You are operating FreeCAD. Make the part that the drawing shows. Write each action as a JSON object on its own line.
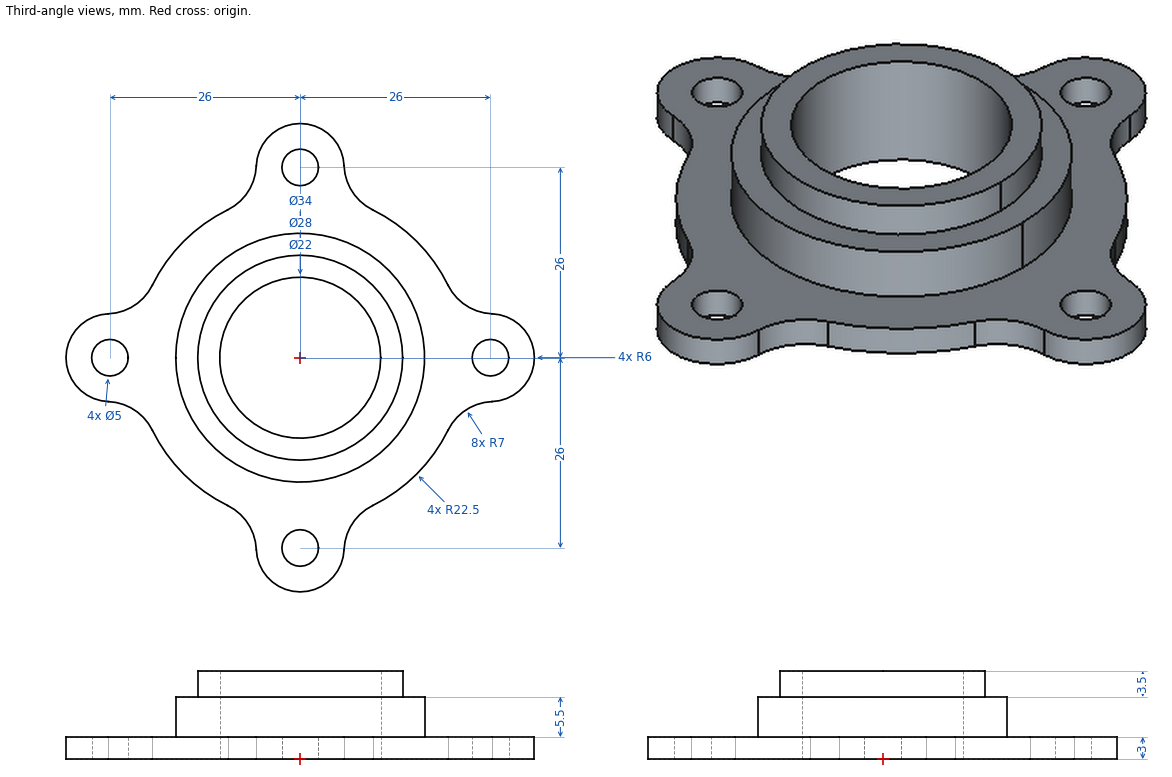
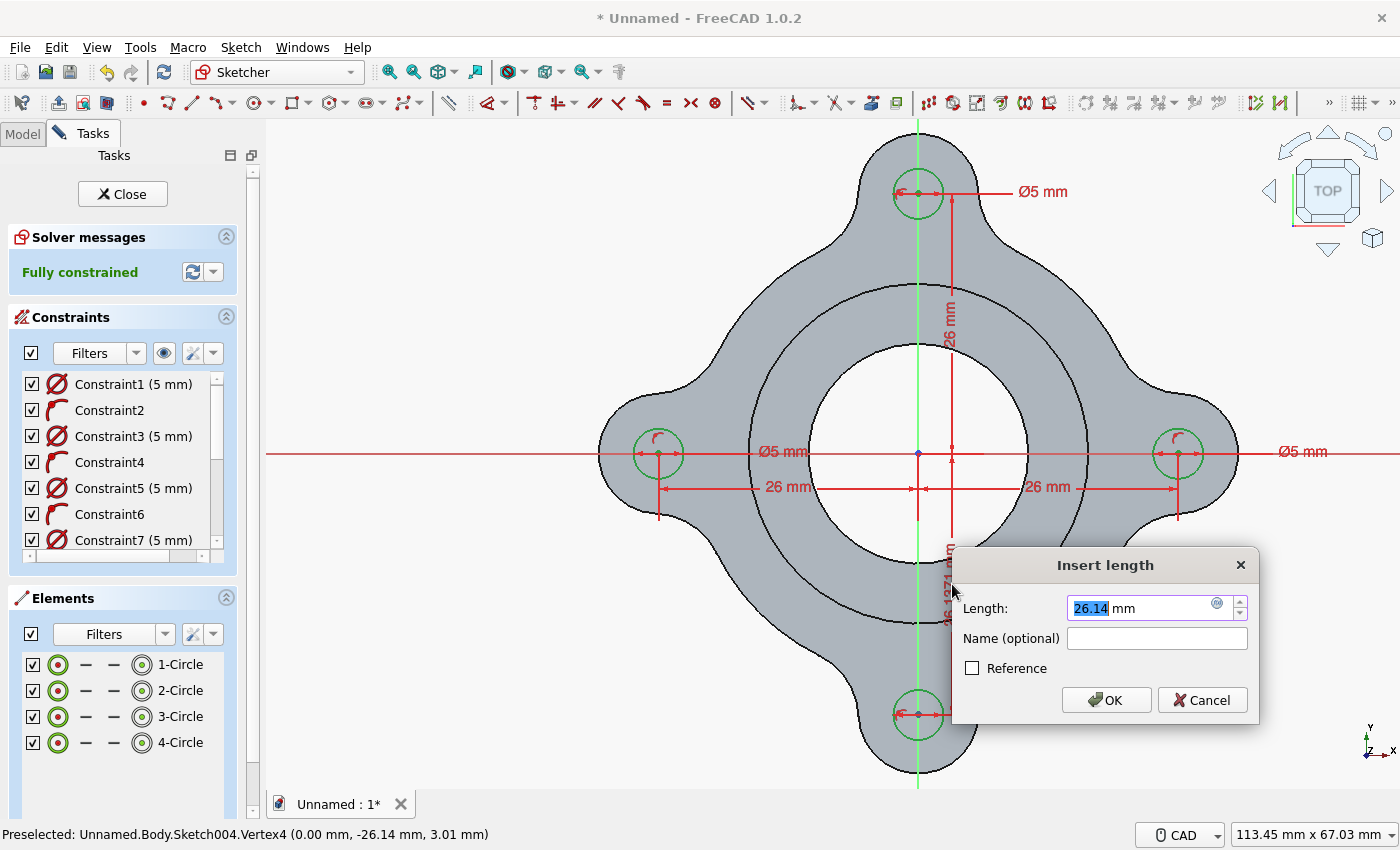
{"action": "type", "text": "26"}
{"action": "key", "text": "Return"}
{"action": "key", "text": "Escape"}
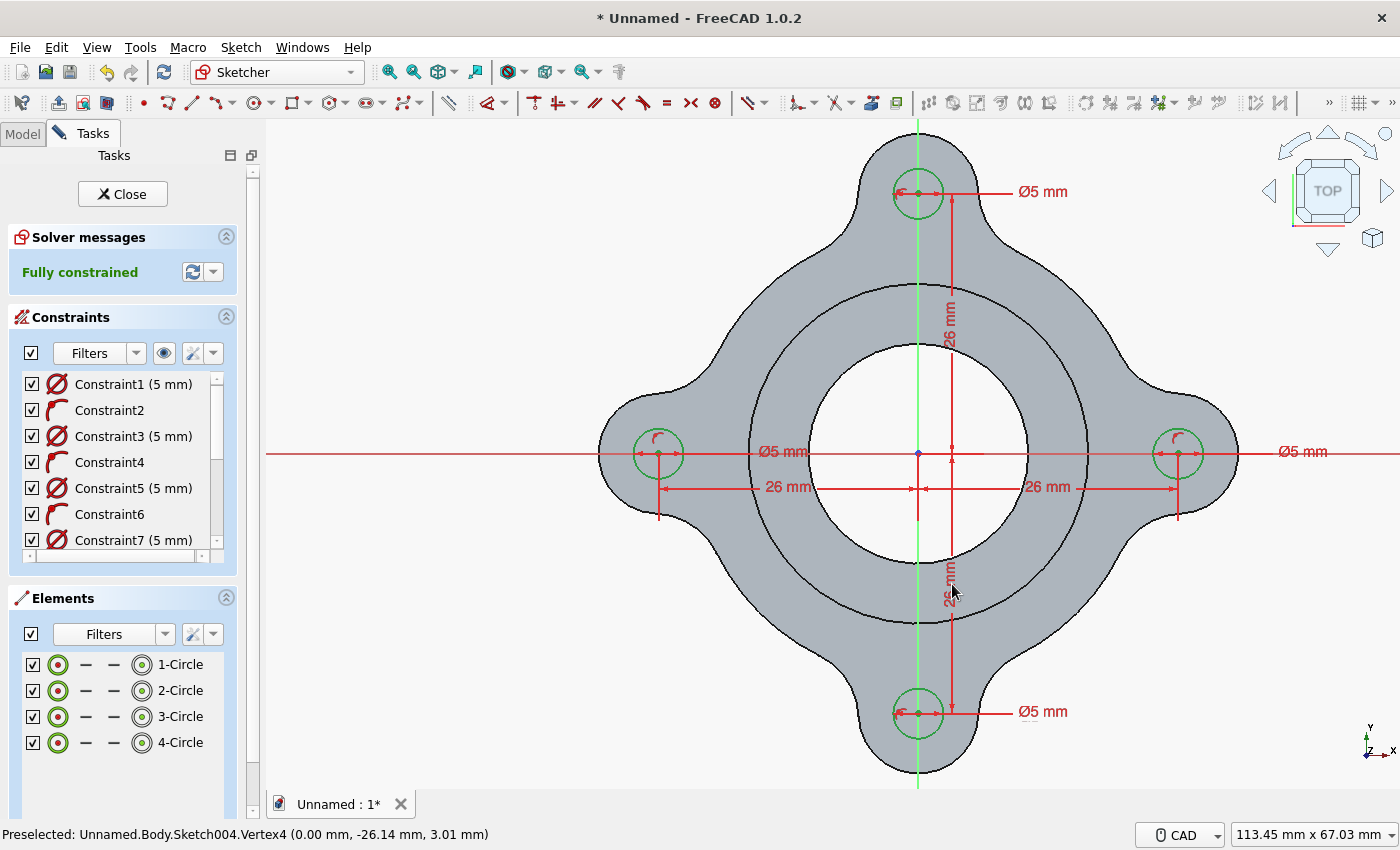
{"action": "left_click", "coordinate": [123, 194]}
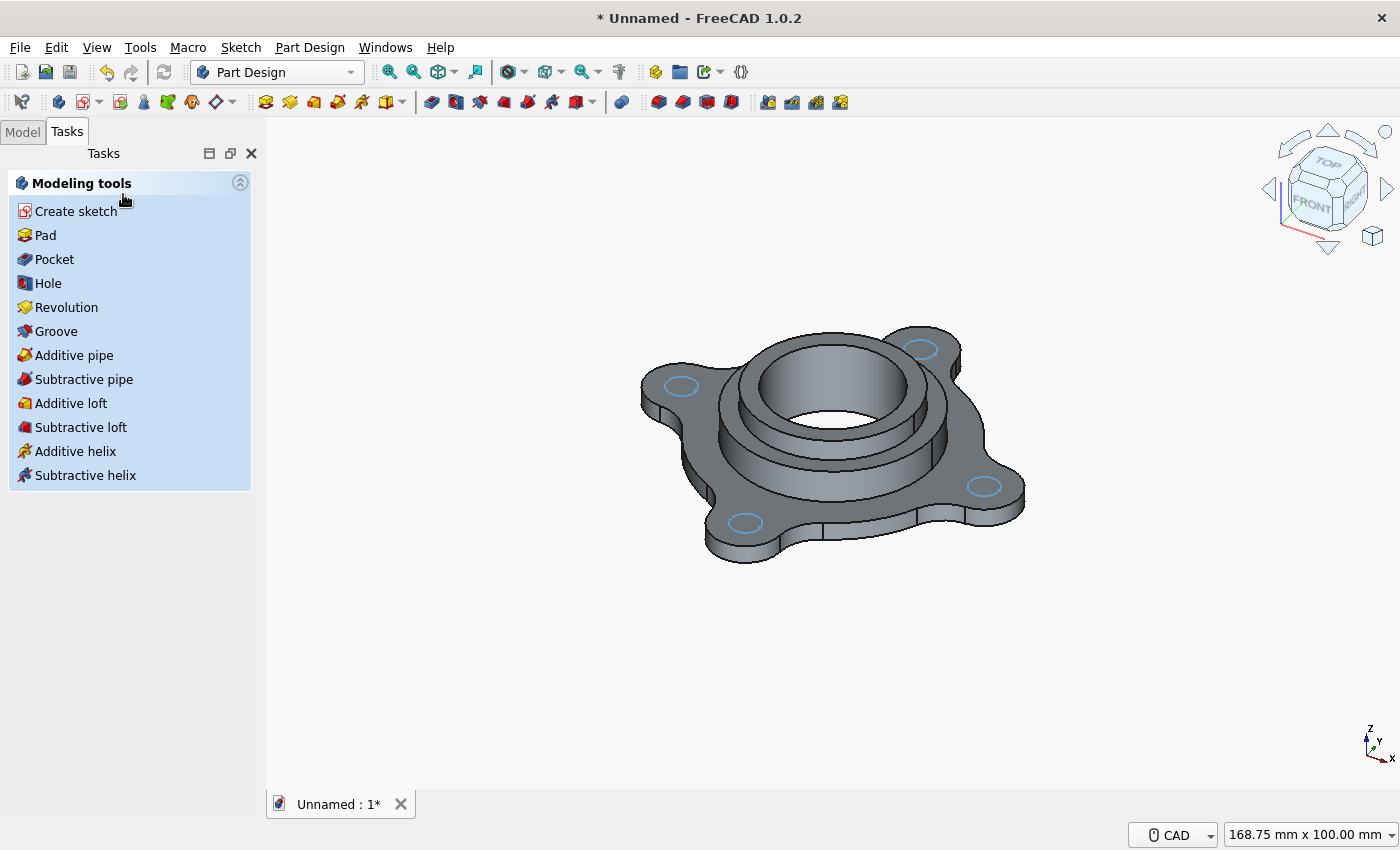
{"action": "left_click", "coordinate": [432, 102]}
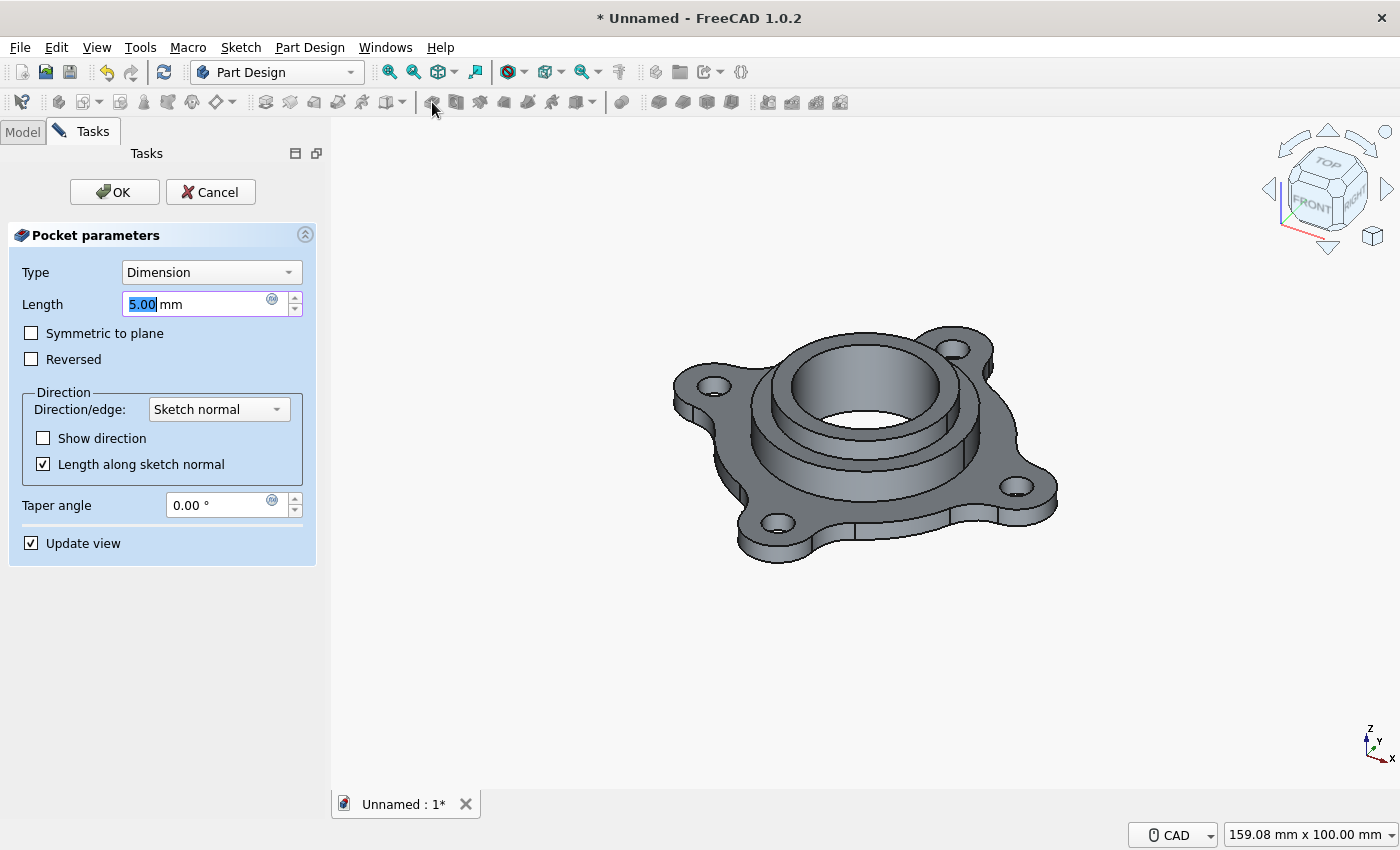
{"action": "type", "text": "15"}
{"action": "key", "text": "Tab"}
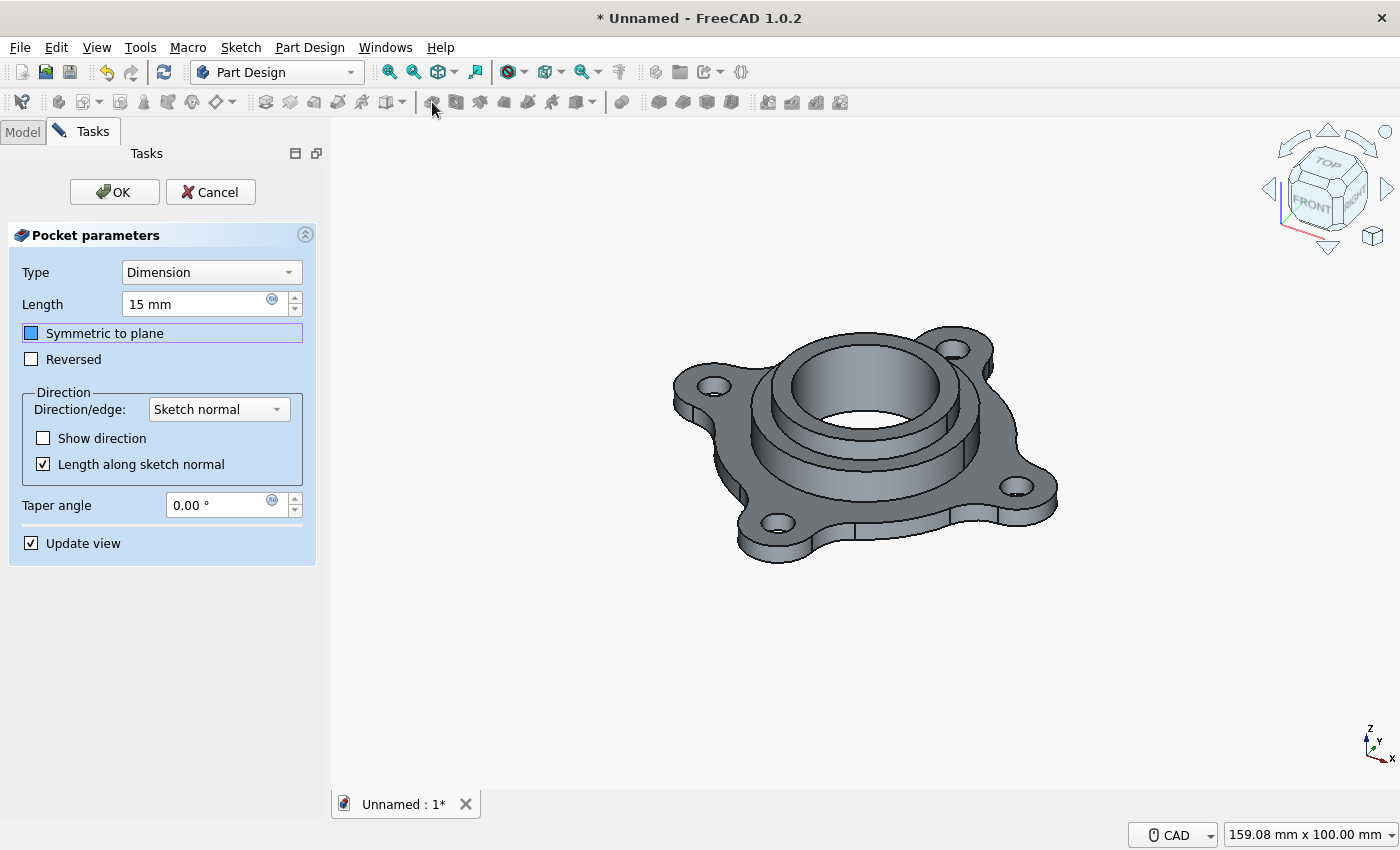
{"action": "left_click", "coordinate": [115, 192]}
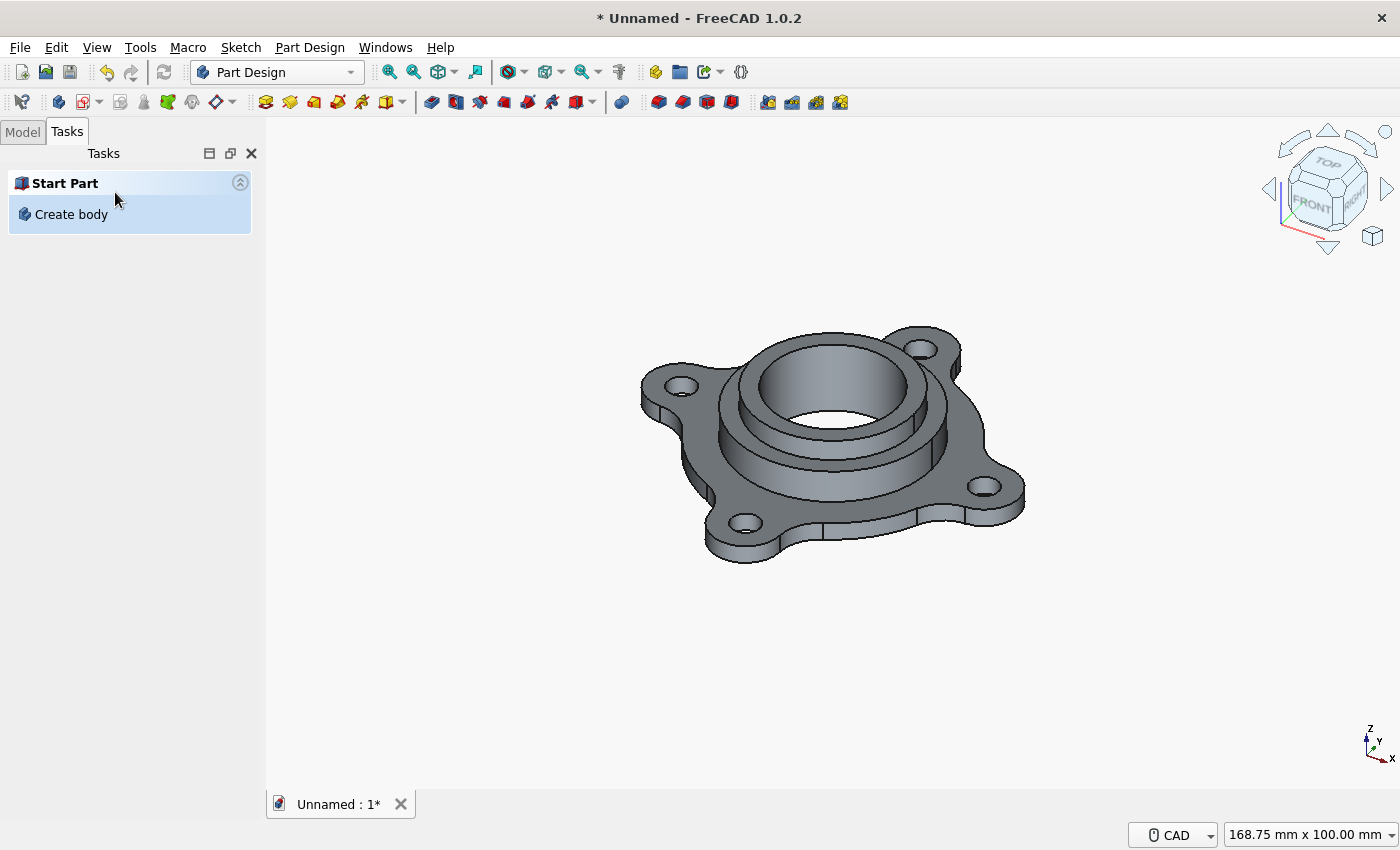
{"action": "key", "text": "0"}